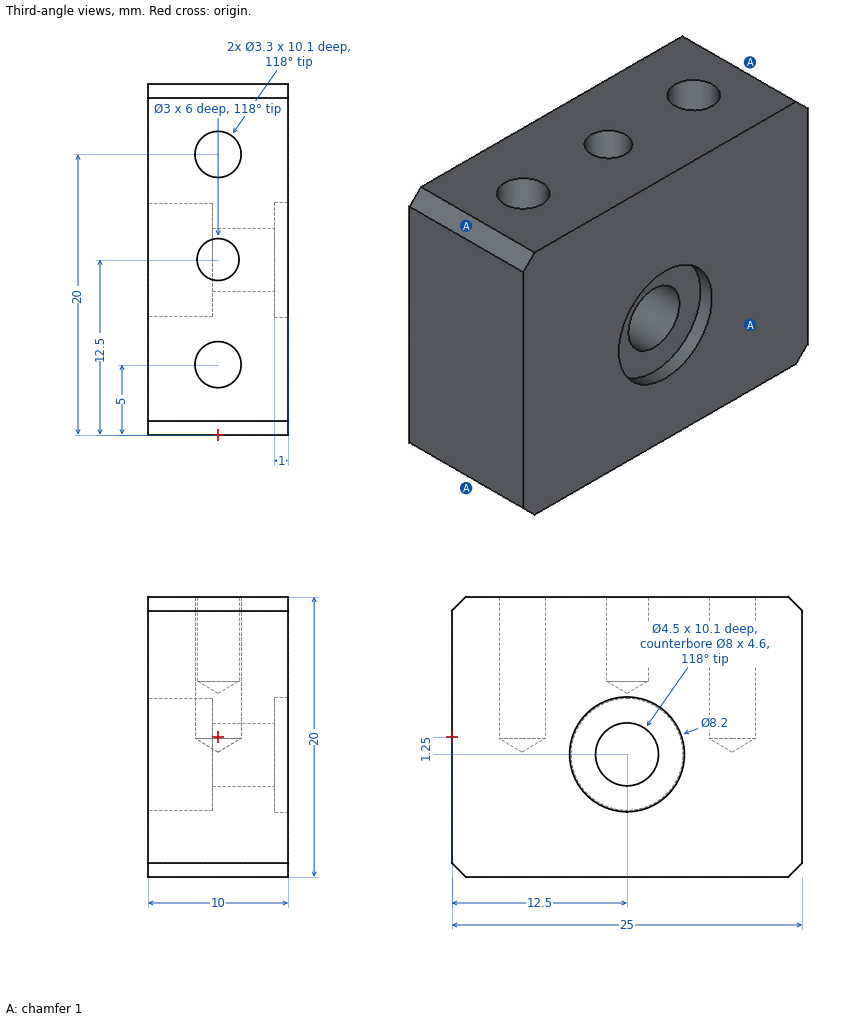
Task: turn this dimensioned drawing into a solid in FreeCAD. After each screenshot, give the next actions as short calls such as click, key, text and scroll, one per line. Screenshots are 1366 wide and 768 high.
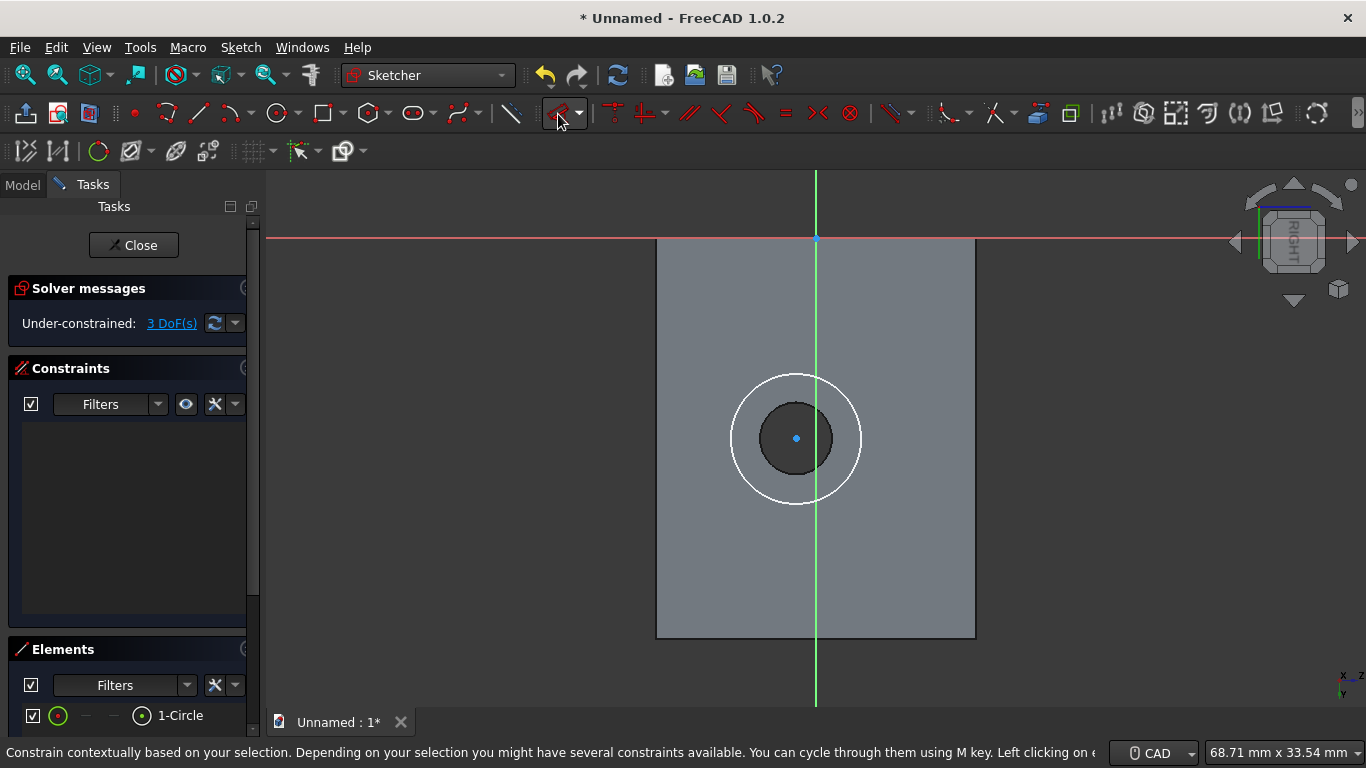
click(842, 393)
click(865, 370)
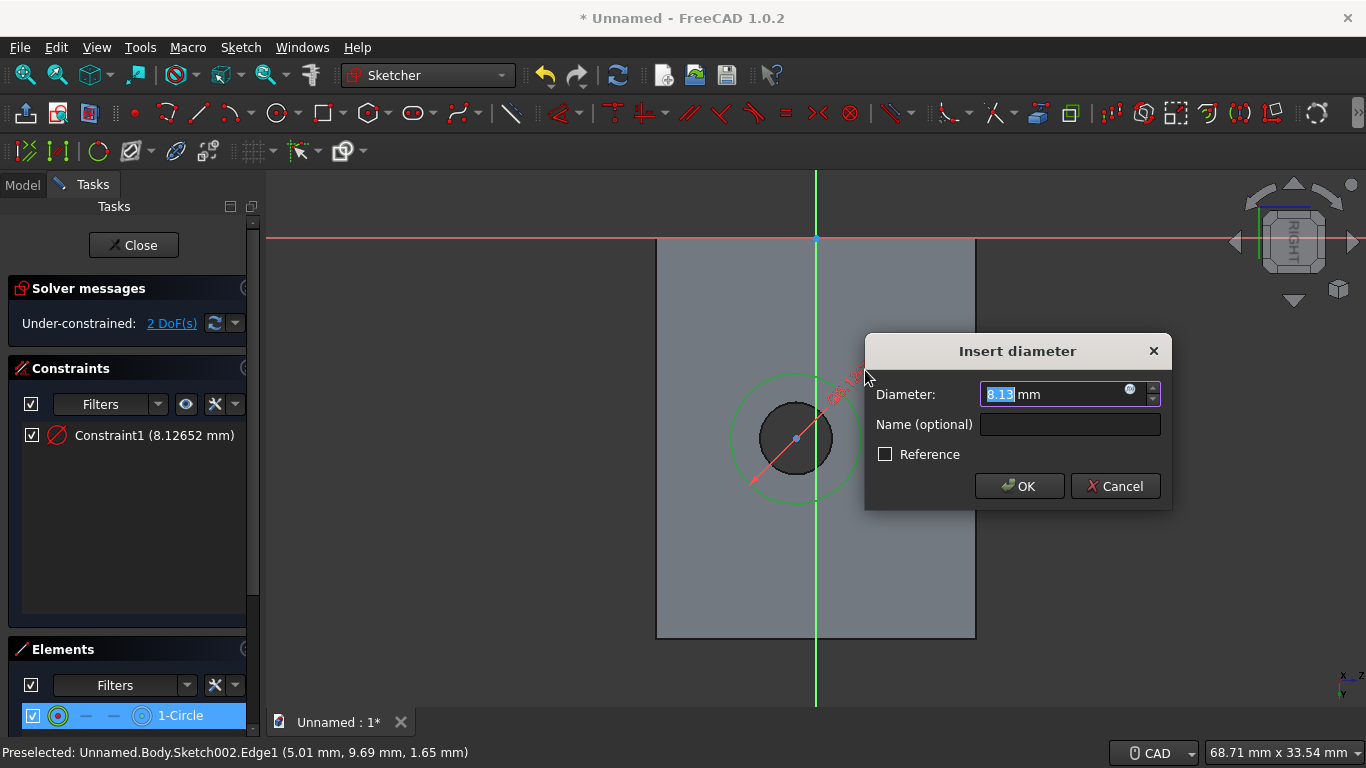
text(8.2)
key(Return)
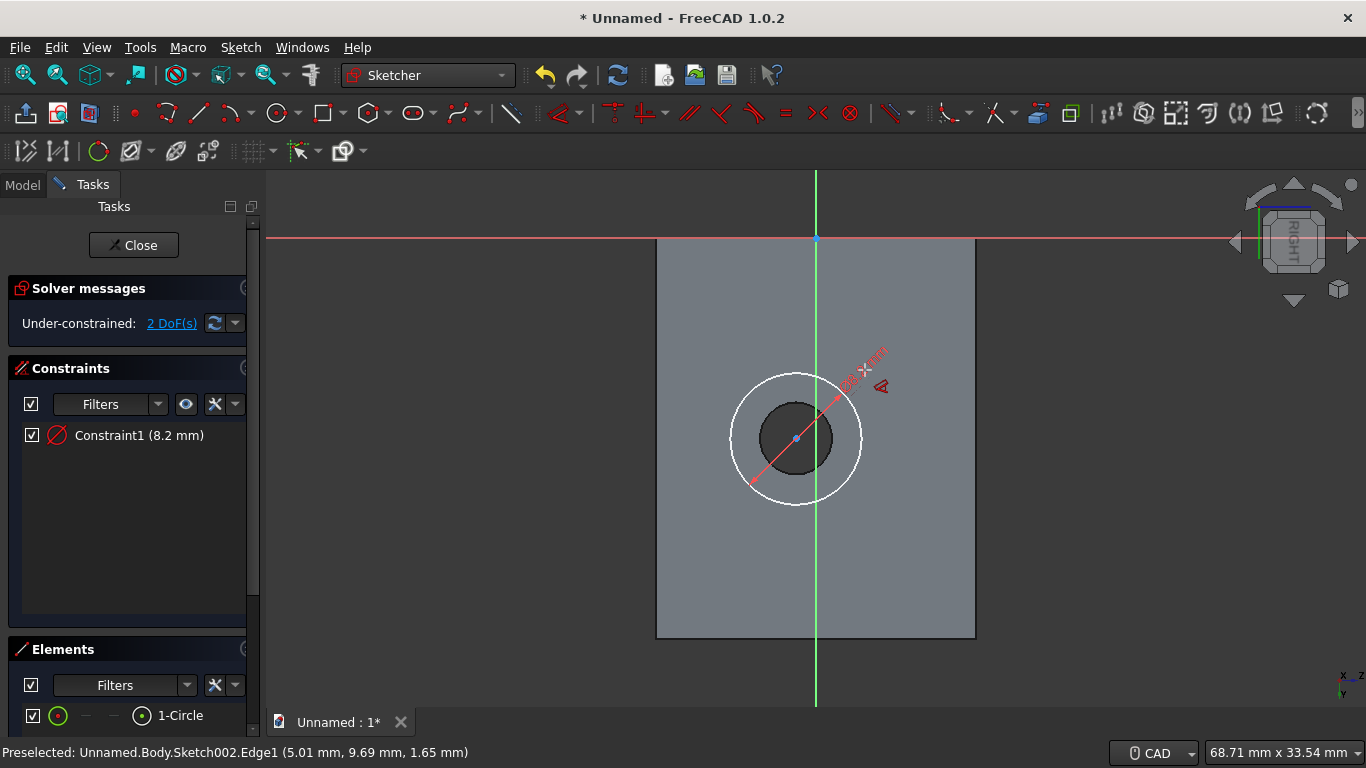
scroll(796, 439, up, 4)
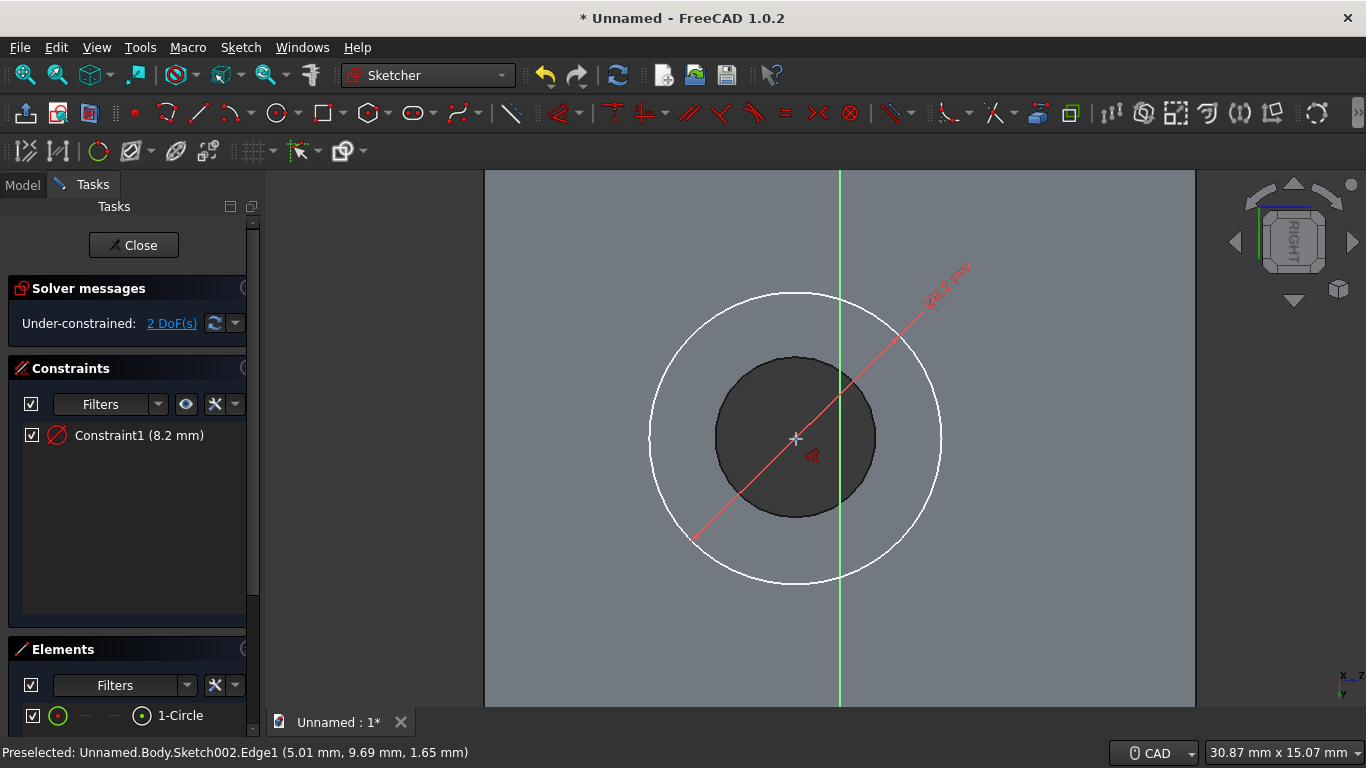
click(795, 438)
click(818, 472)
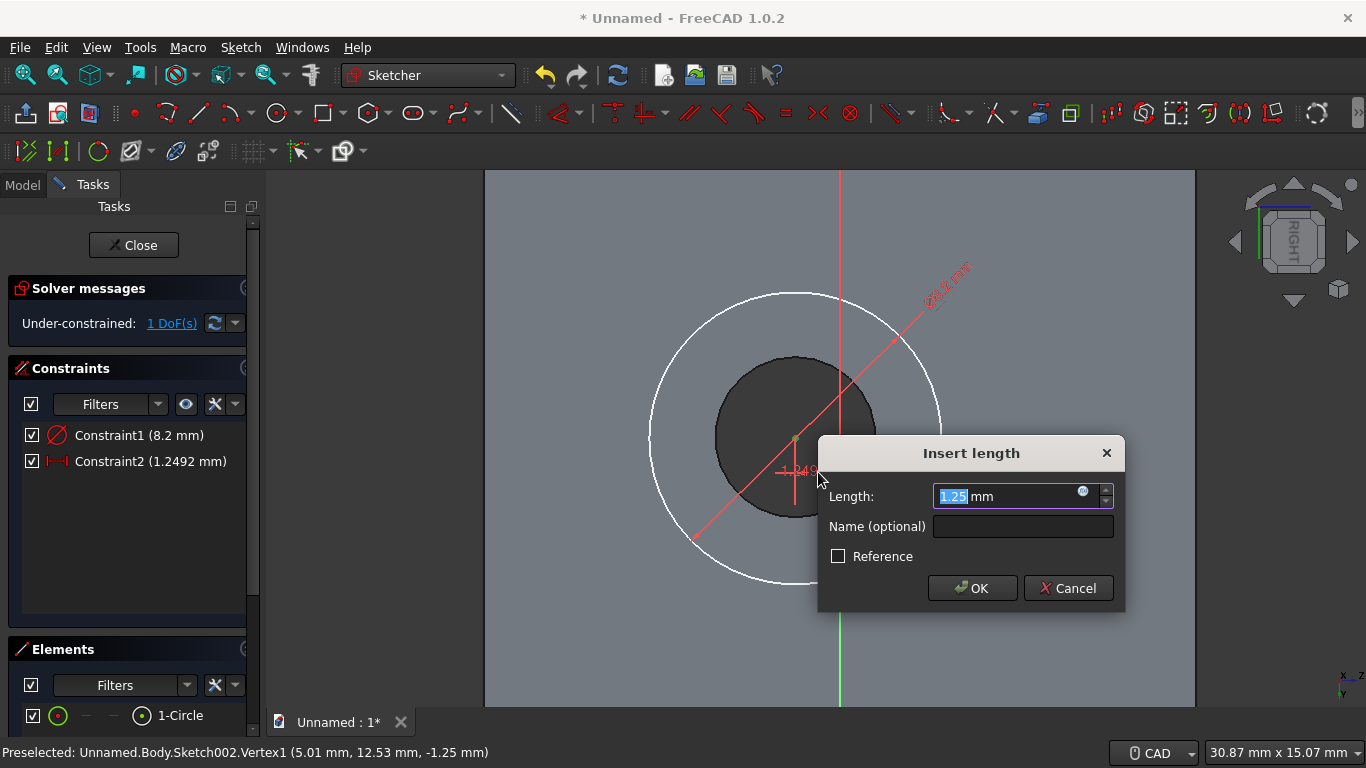
text(1.25)
key(Return)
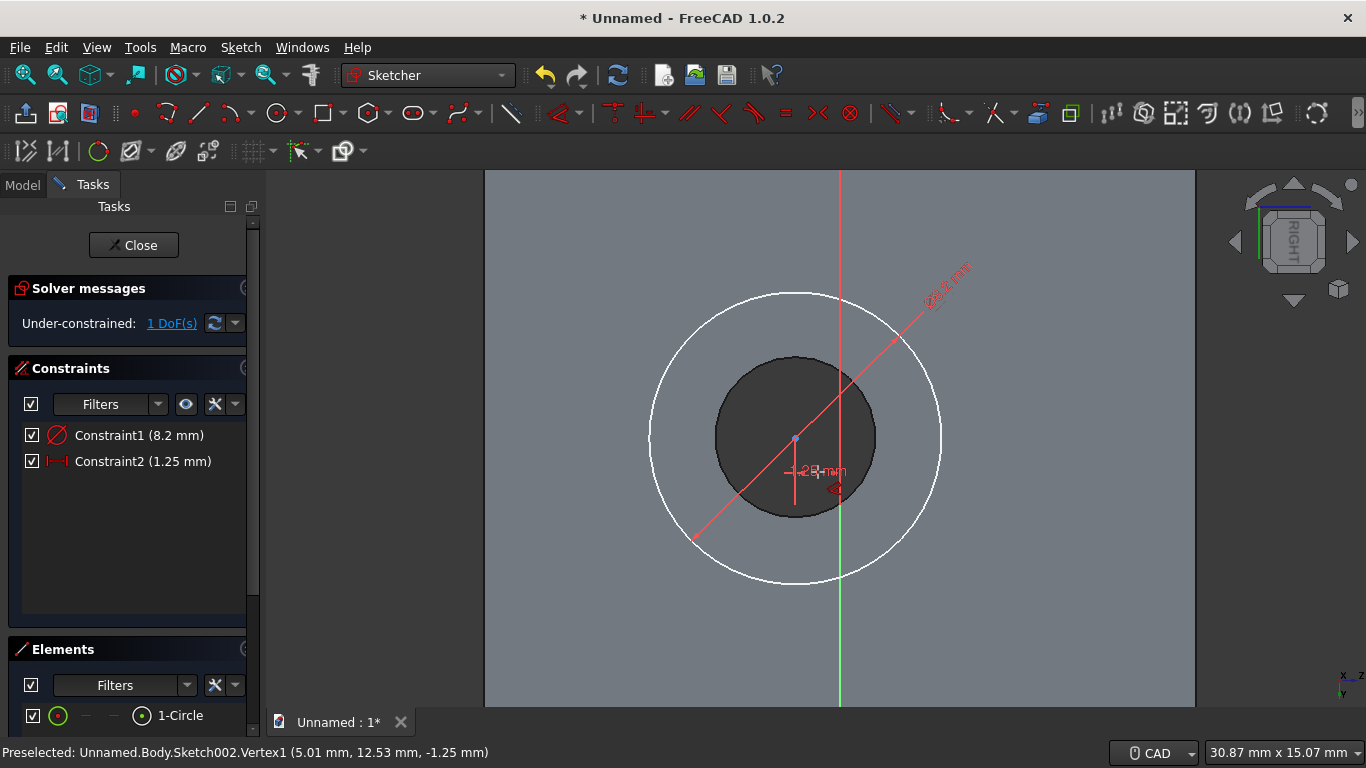
click(795, 438)
click(874, 263)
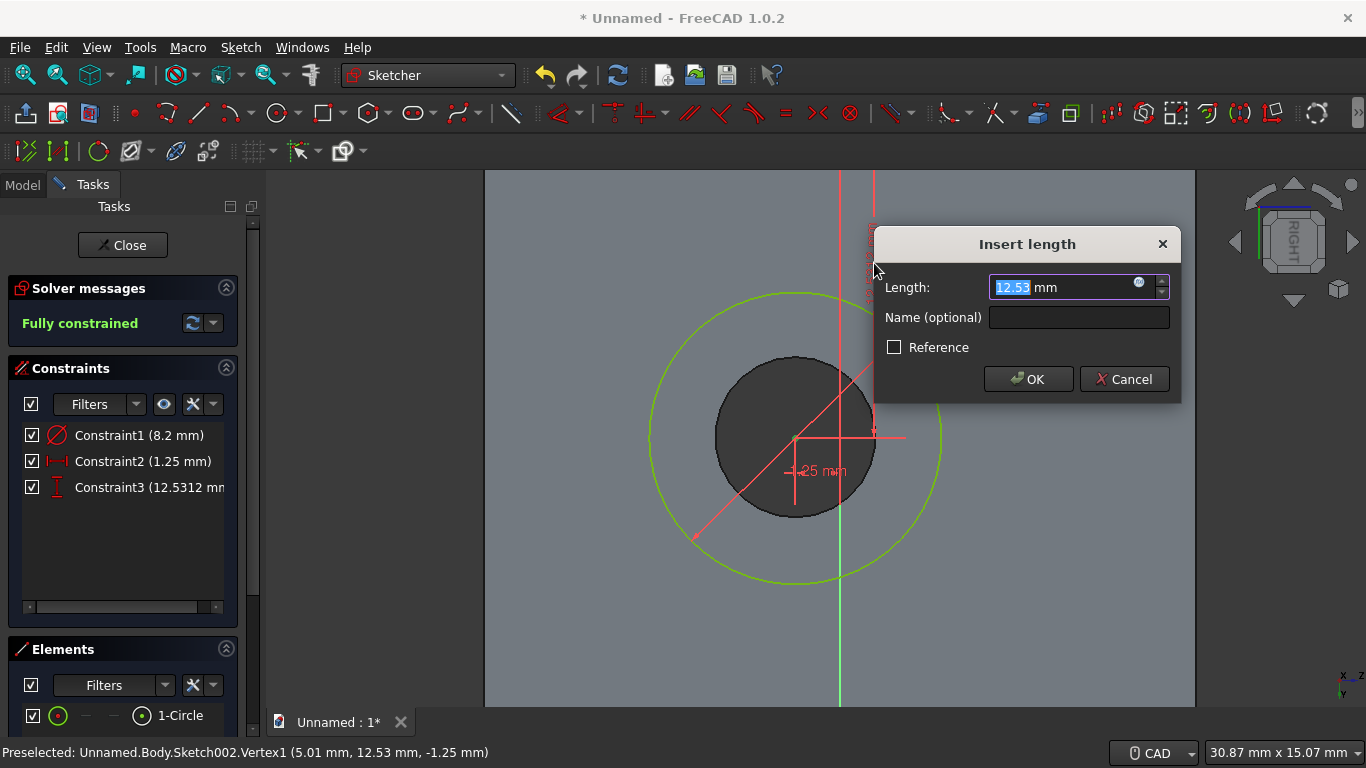
text(12.5)
key(Return)
key(Escape)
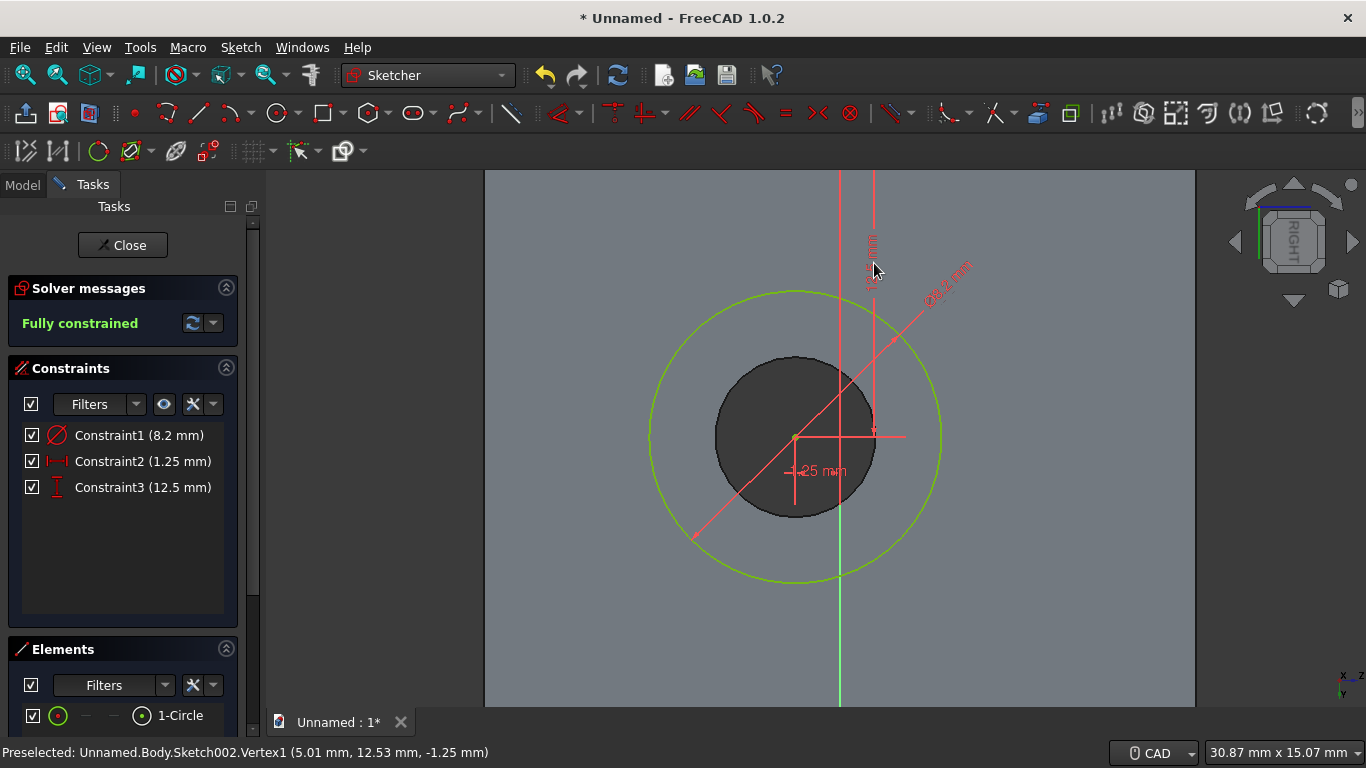
click(123, 245)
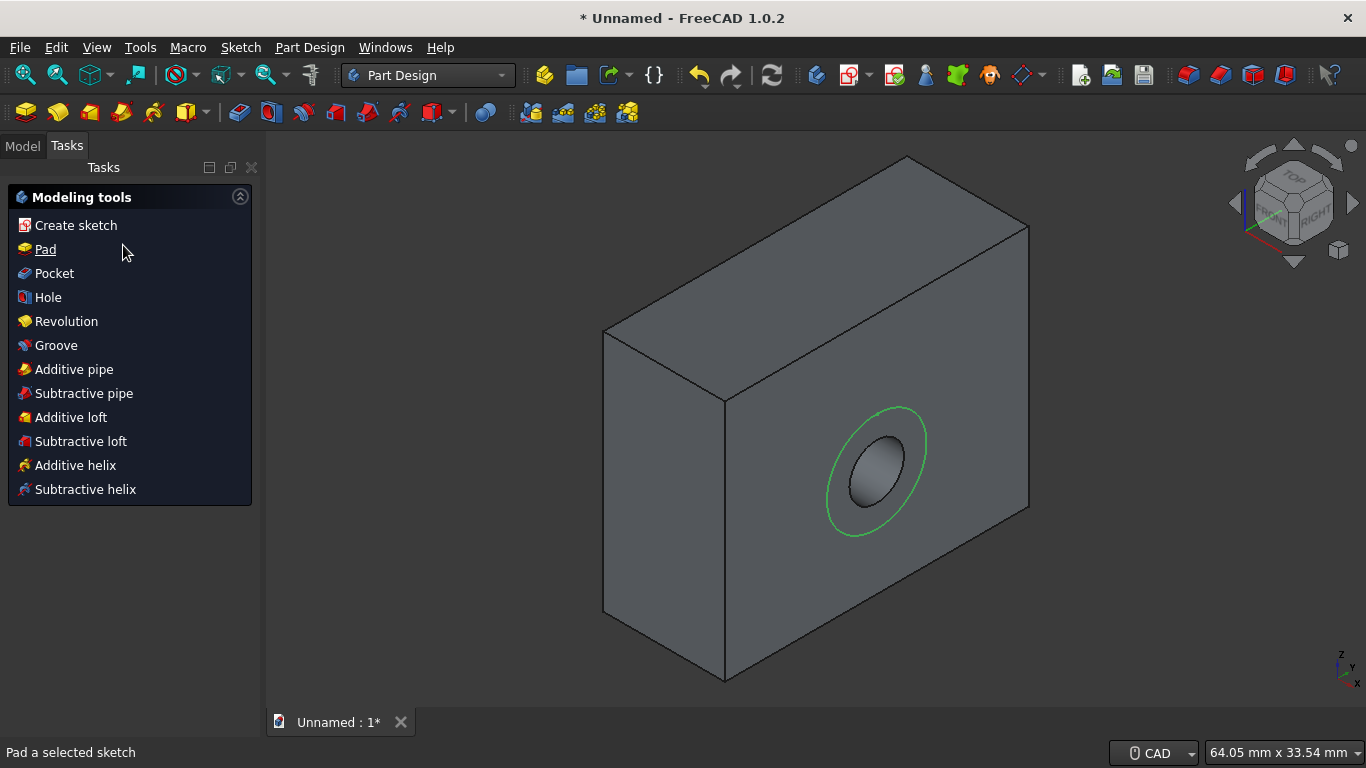
click(240, 112)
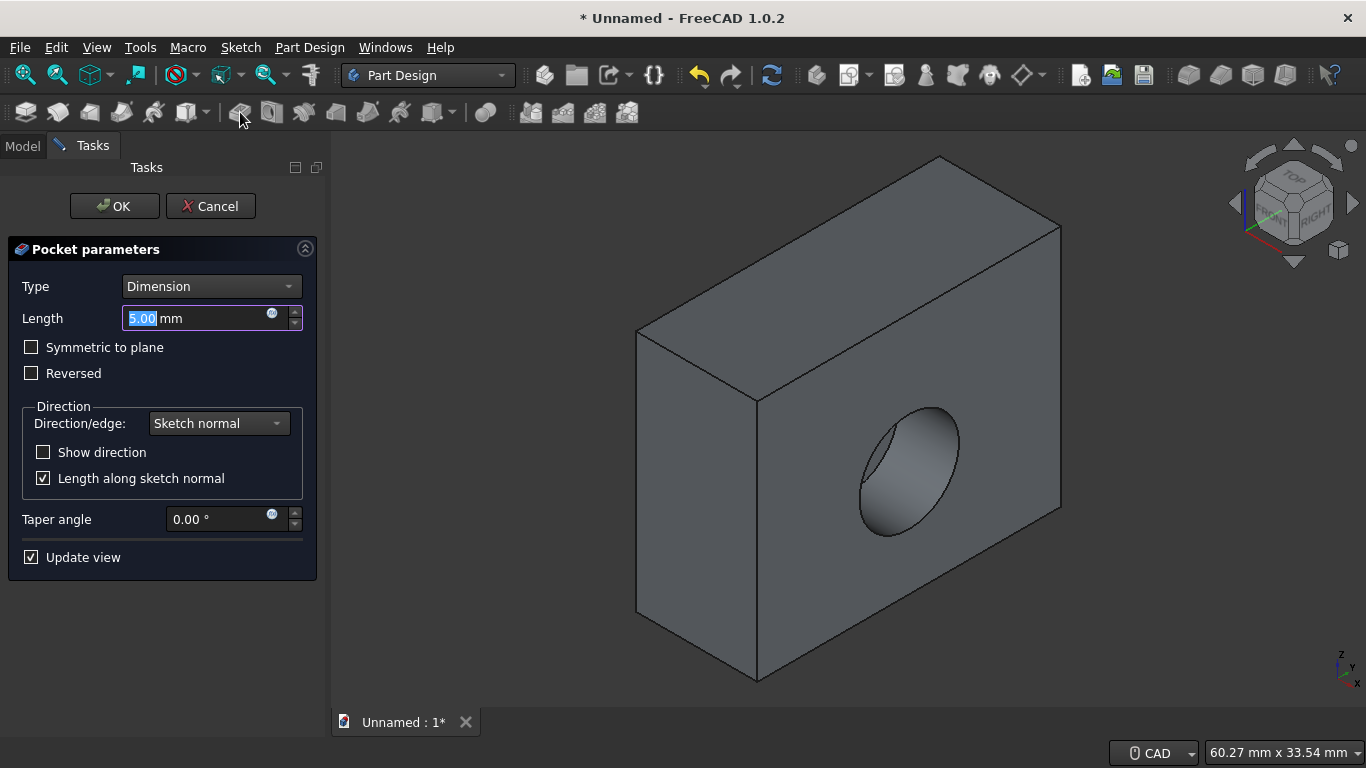
text(1)
key(Tab)